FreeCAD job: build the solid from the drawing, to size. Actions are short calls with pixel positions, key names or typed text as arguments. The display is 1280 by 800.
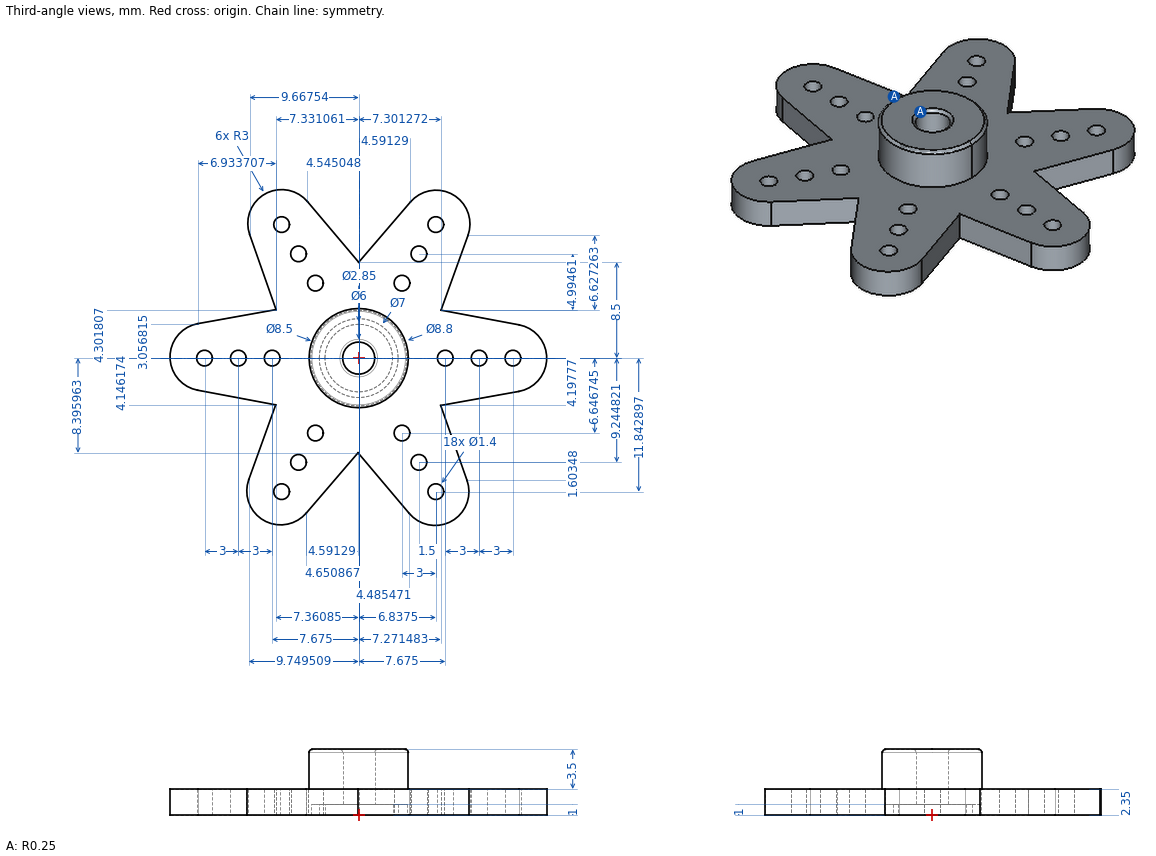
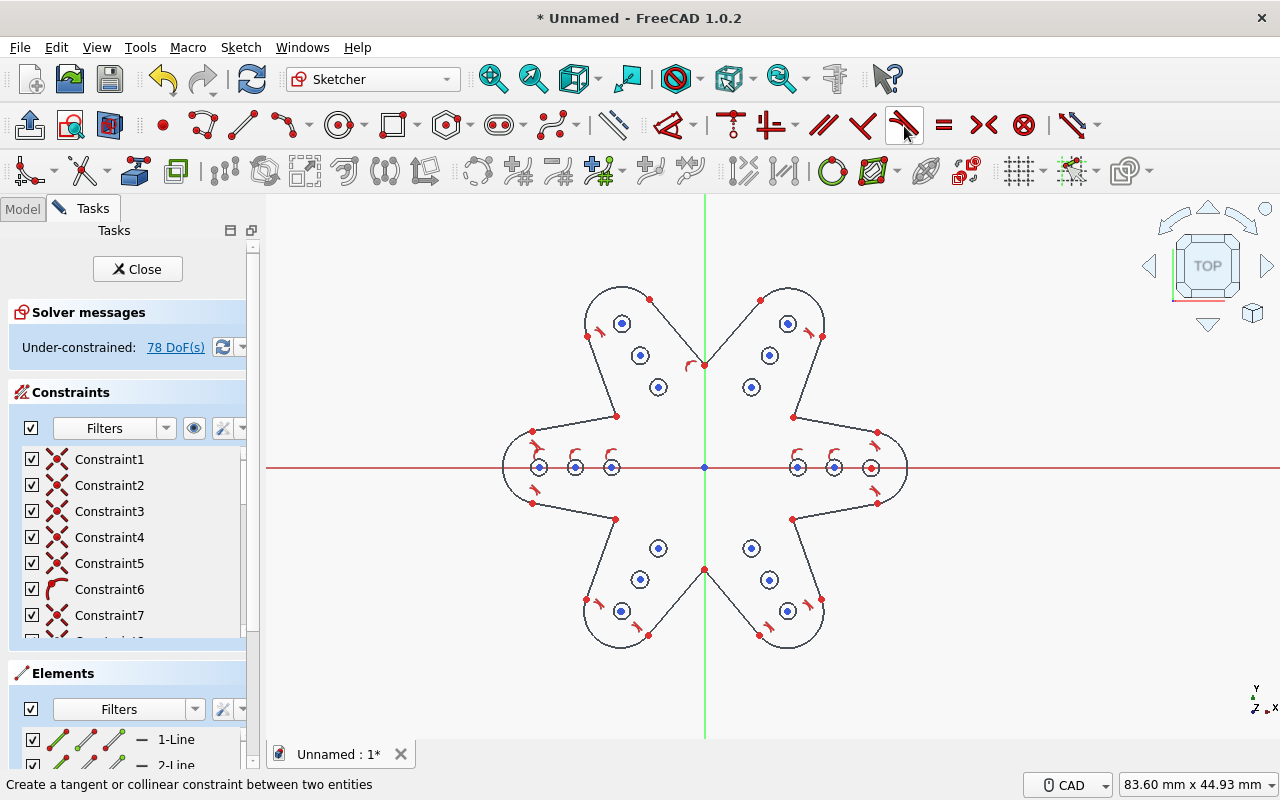
click(744, 320)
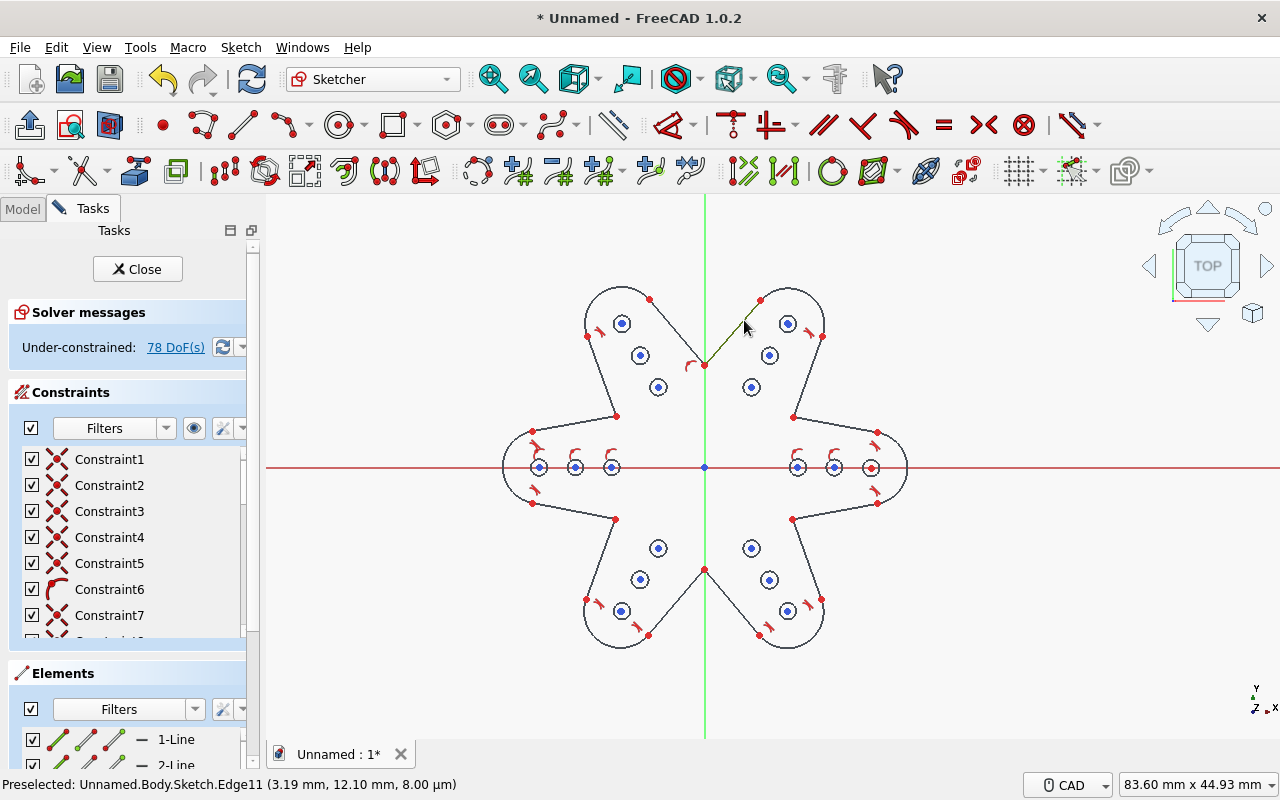
click(820, 308)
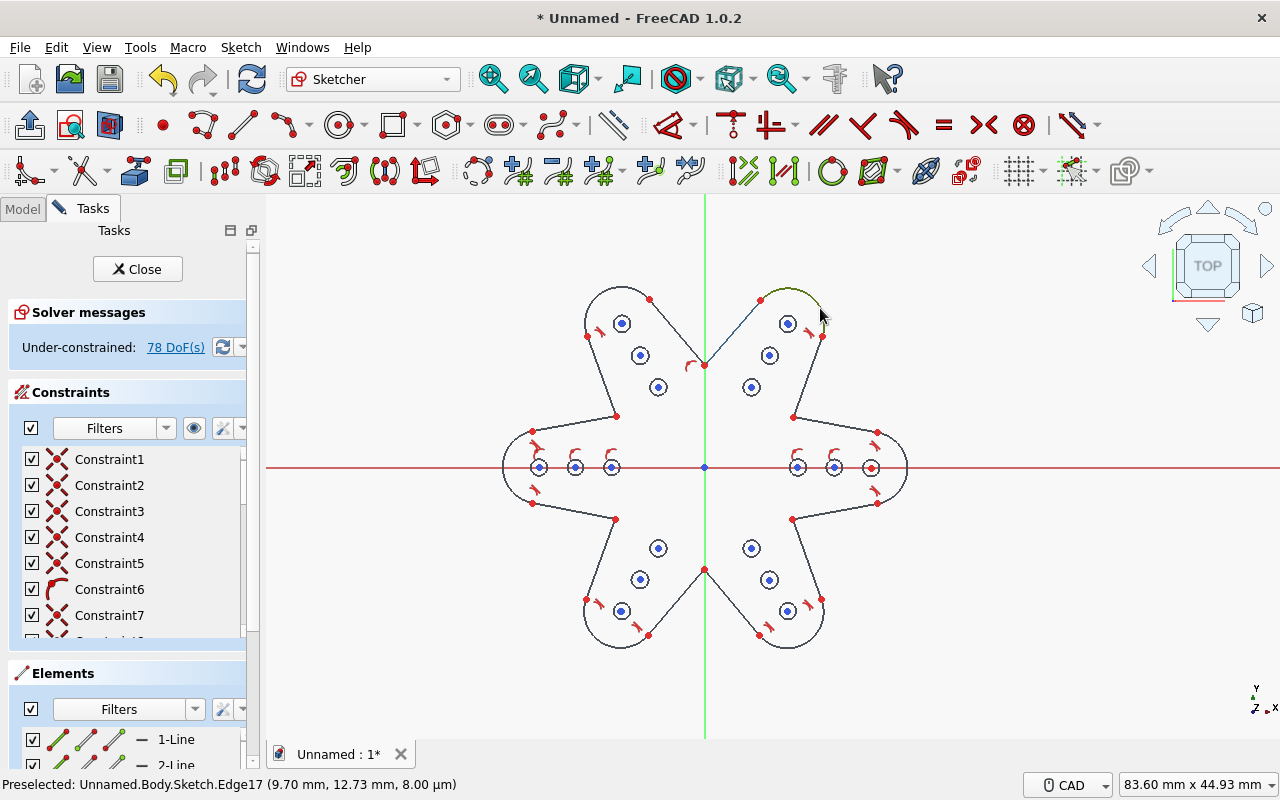
click(904, 126)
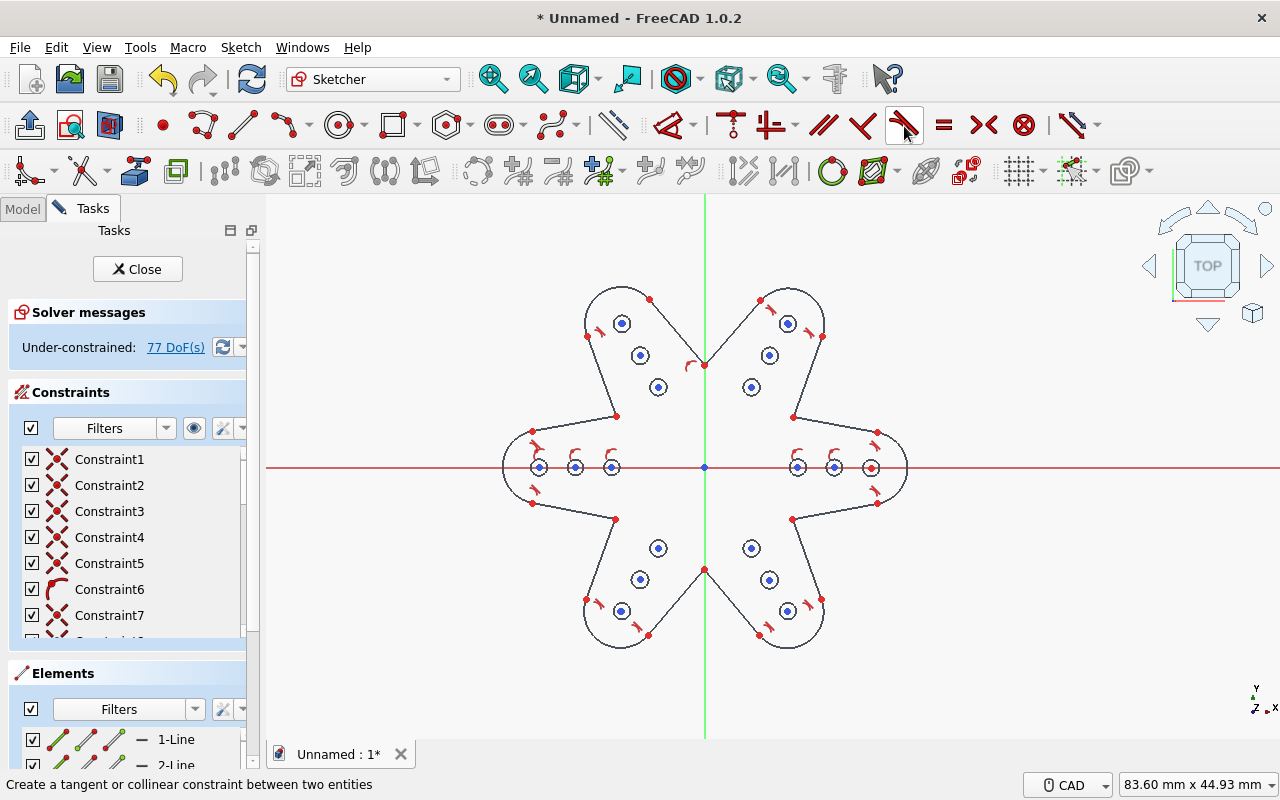
click(688, 346)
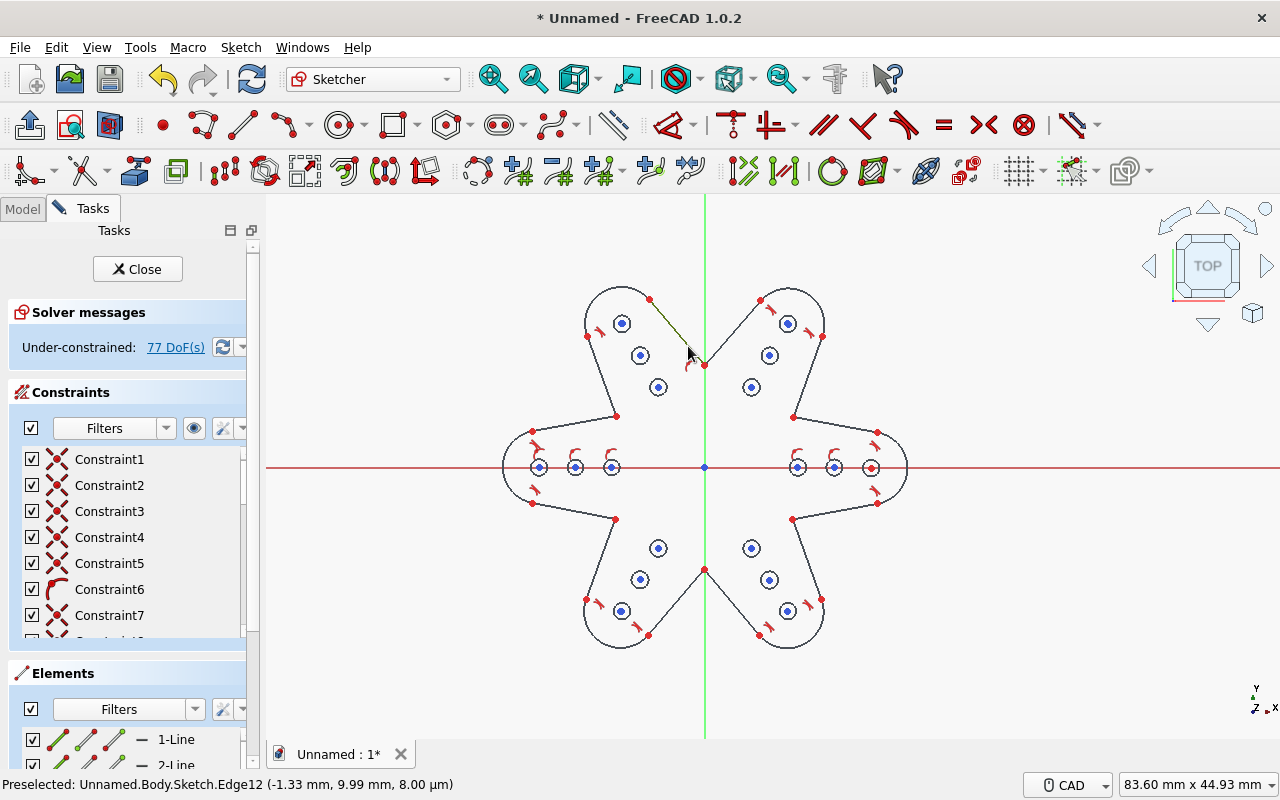
click(623, 287)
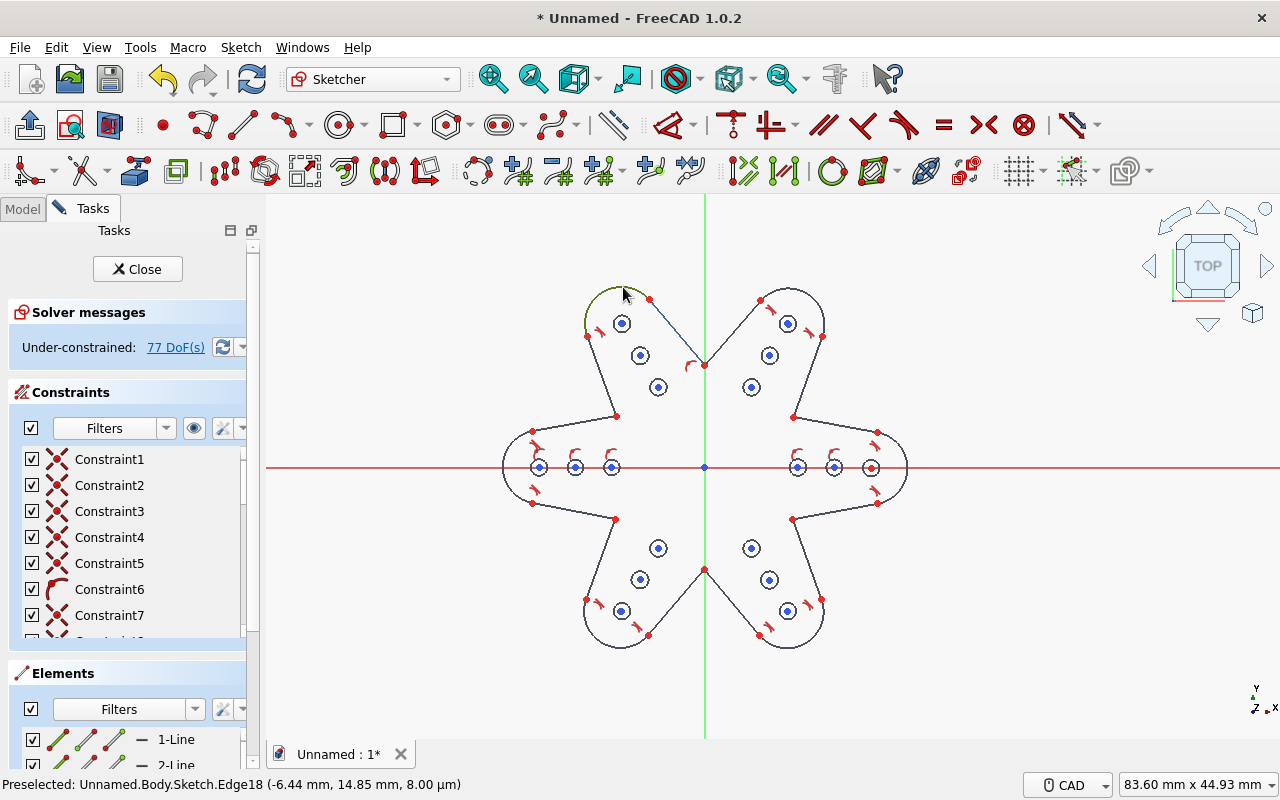
click(904, 126)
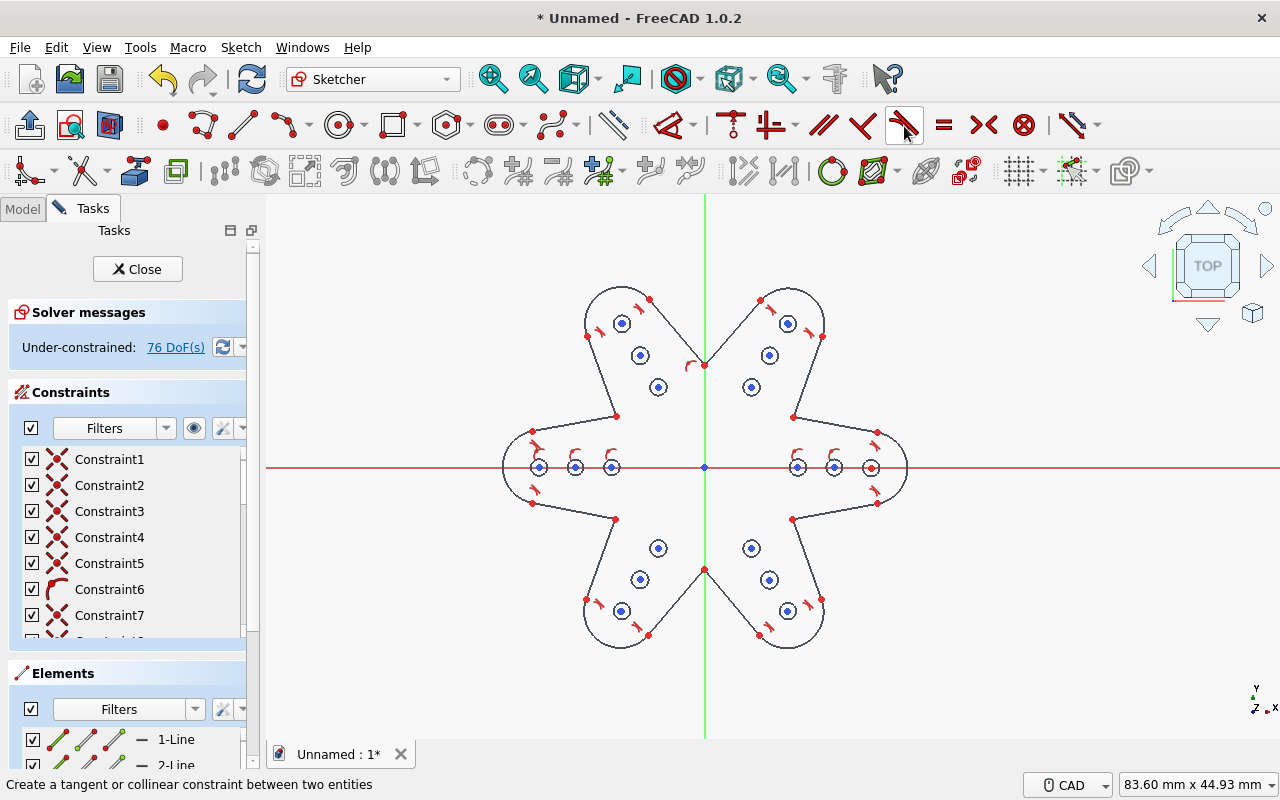
click(508, 448)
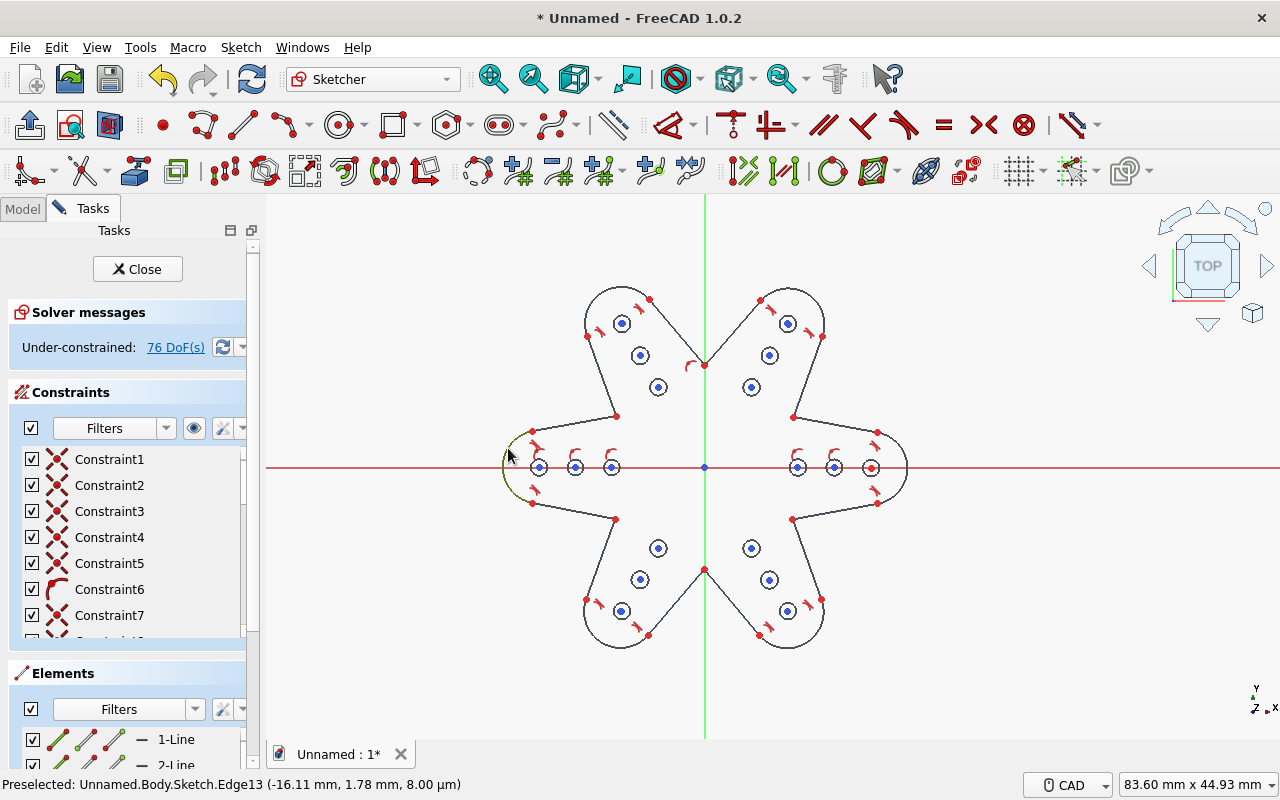
click(588, 629)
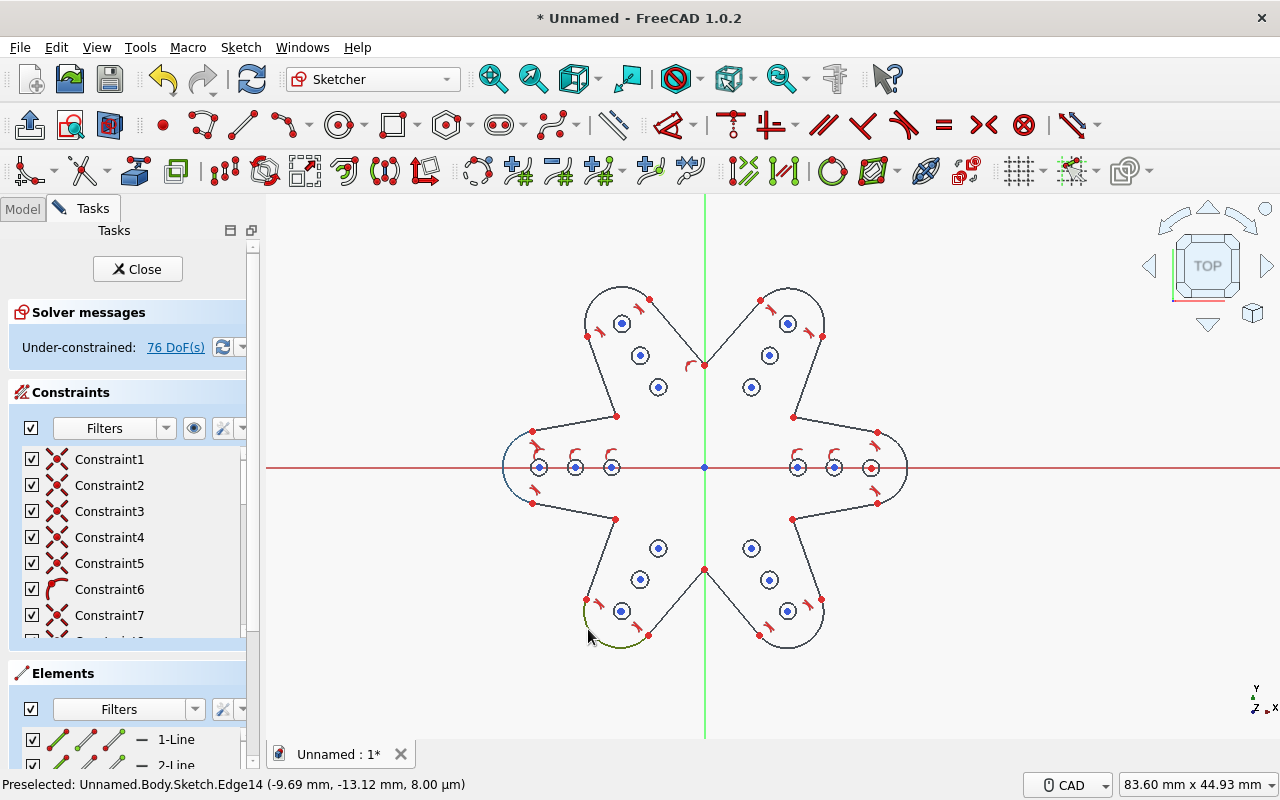
click(786, 648)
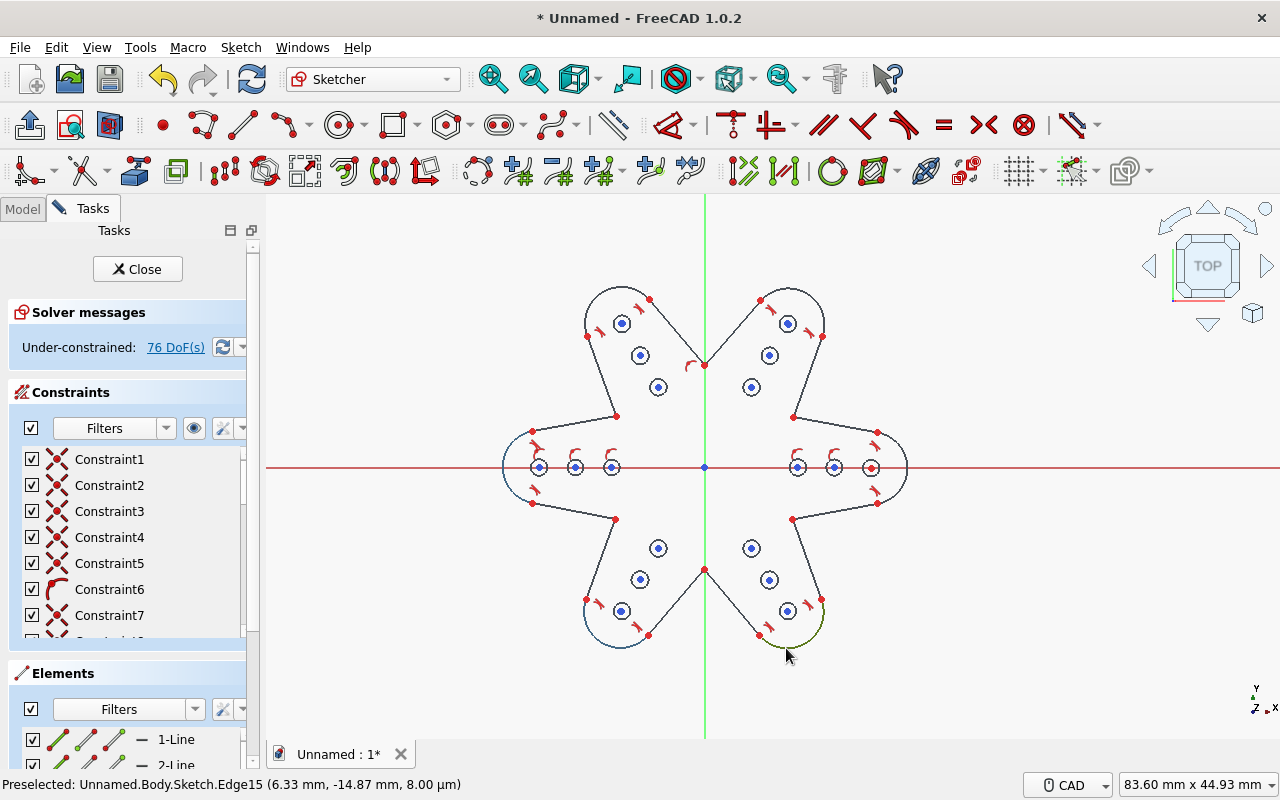
click(902, 487)